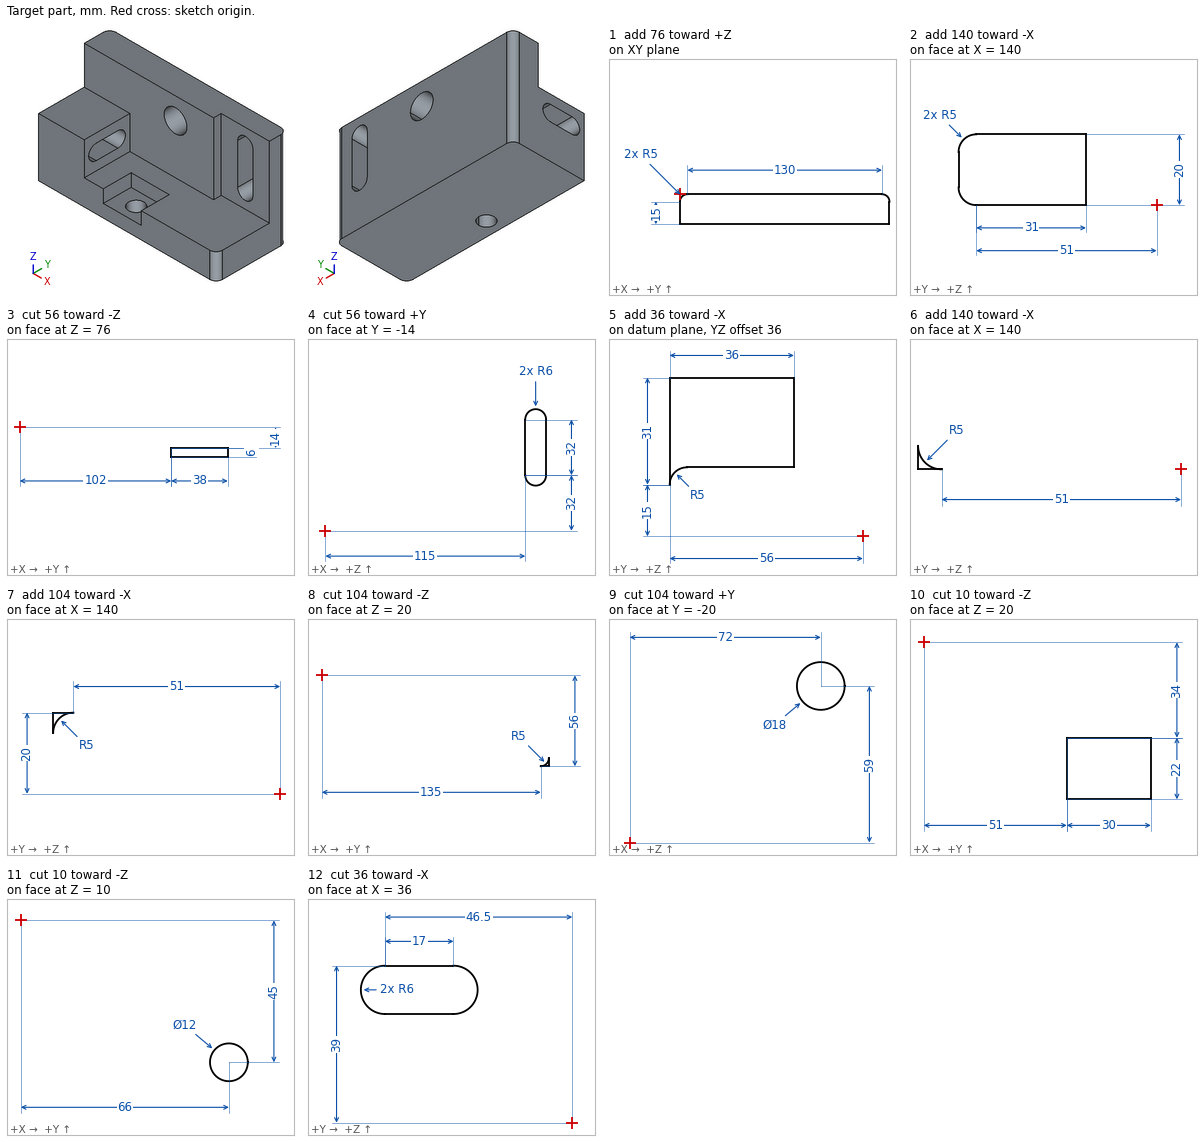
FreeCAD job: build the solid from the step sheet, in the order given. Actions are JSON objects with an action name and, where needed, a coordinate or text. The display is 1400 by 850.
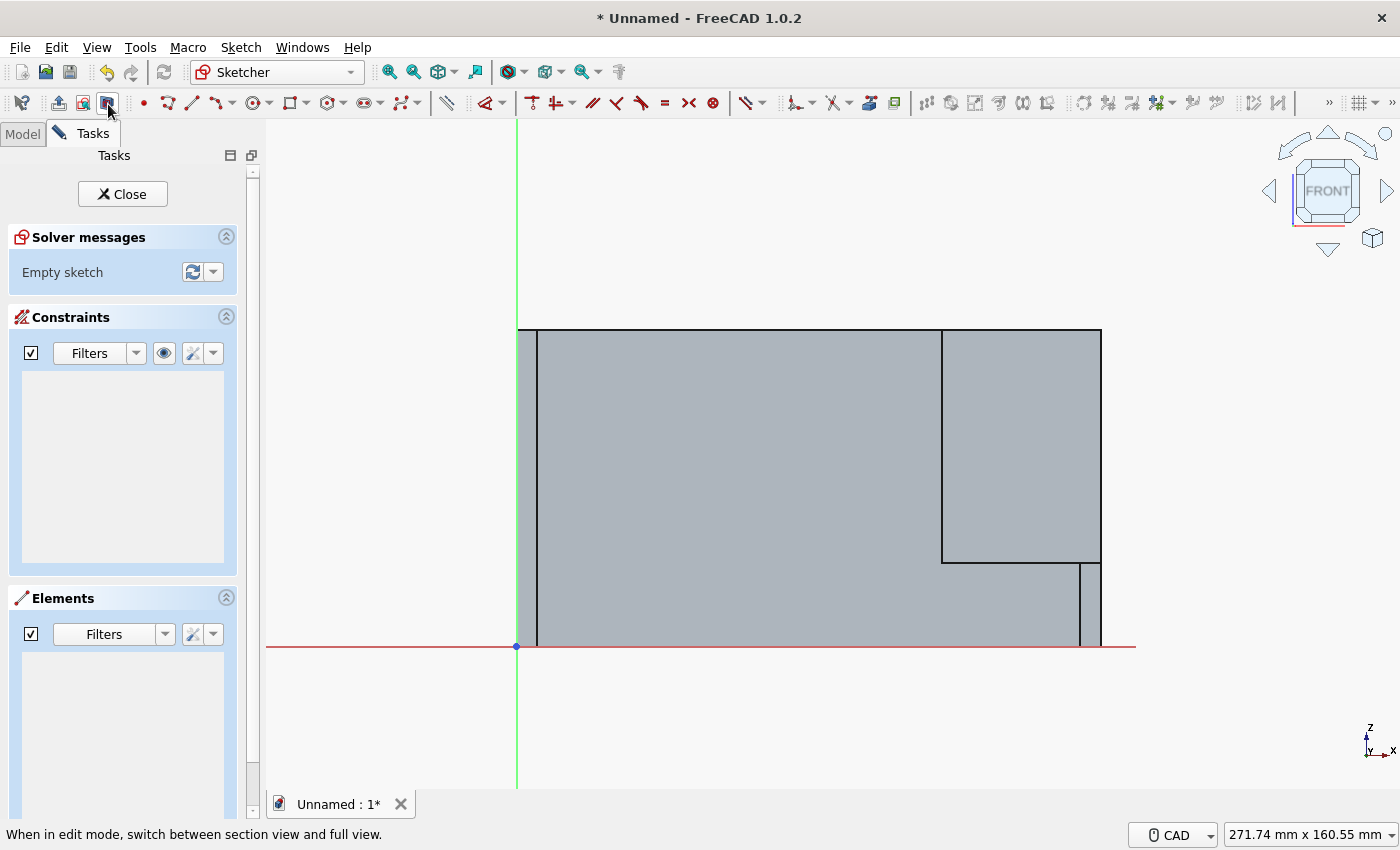
{"action": "scroll", "coordinate": [1231, 440], "scroll_direction": "up", "scroll_amount": 4}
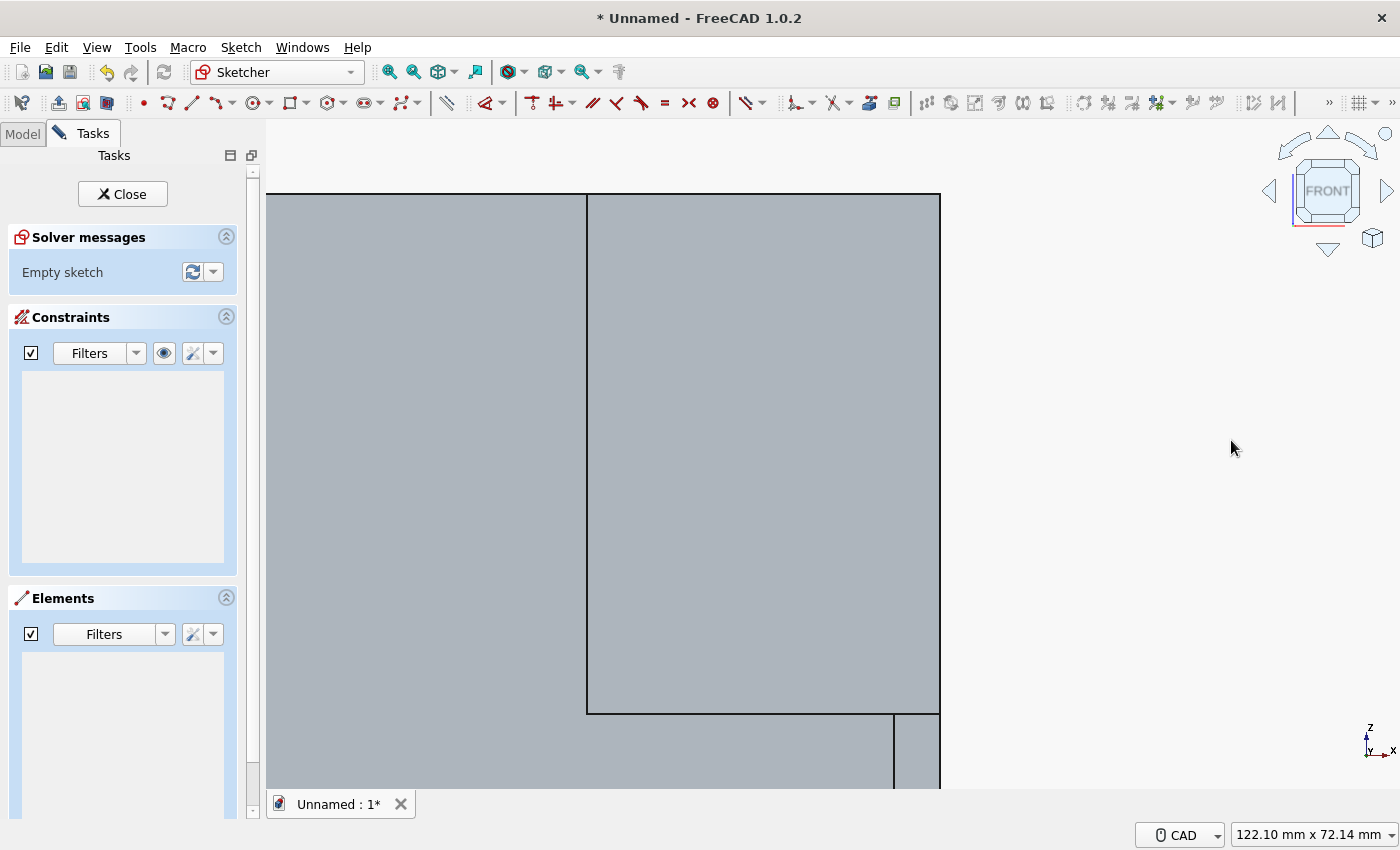
{"action": "left_click", "coordinate": [364, 104]}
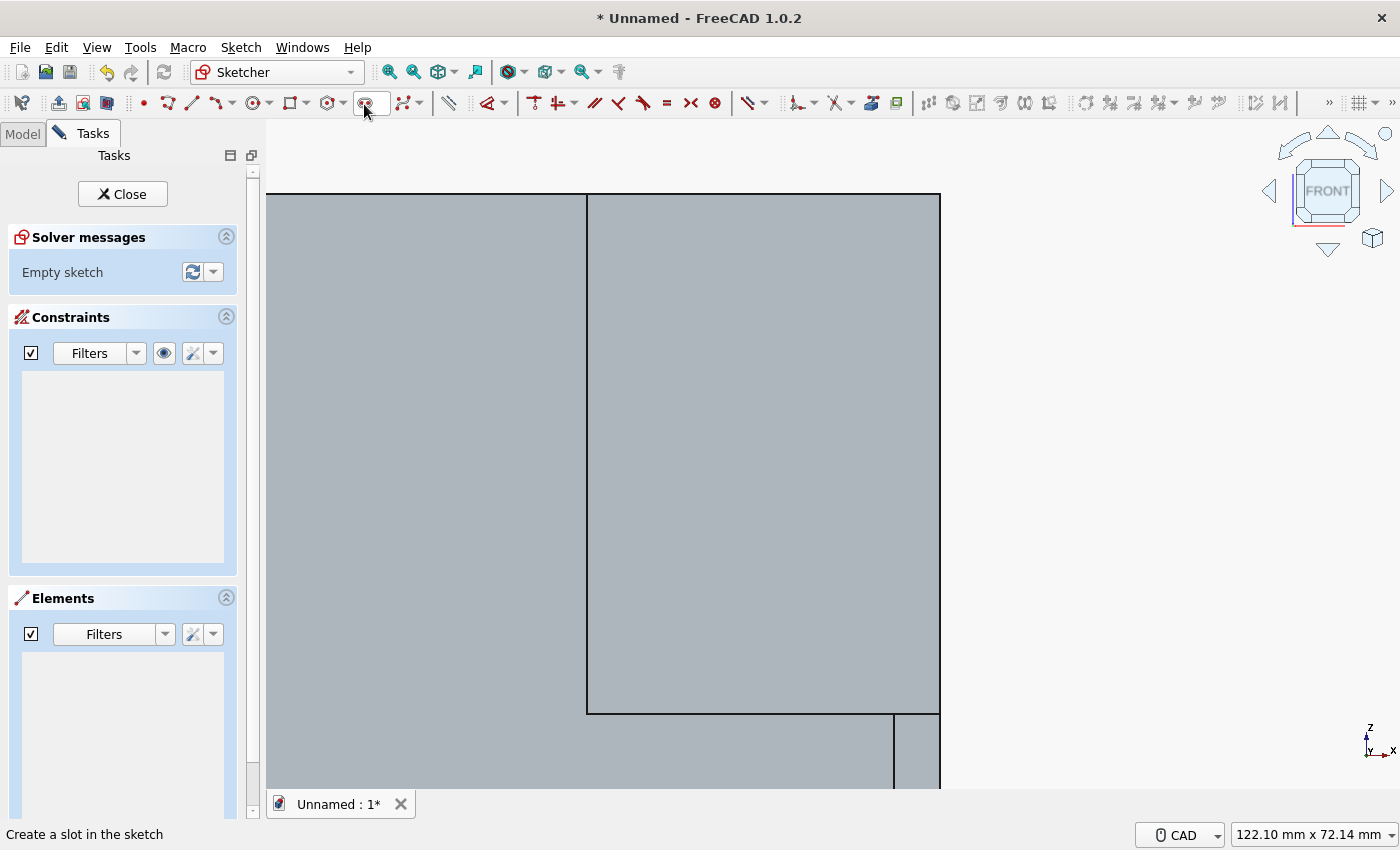
{"action": "left_click", "coordinate": [764, 602]}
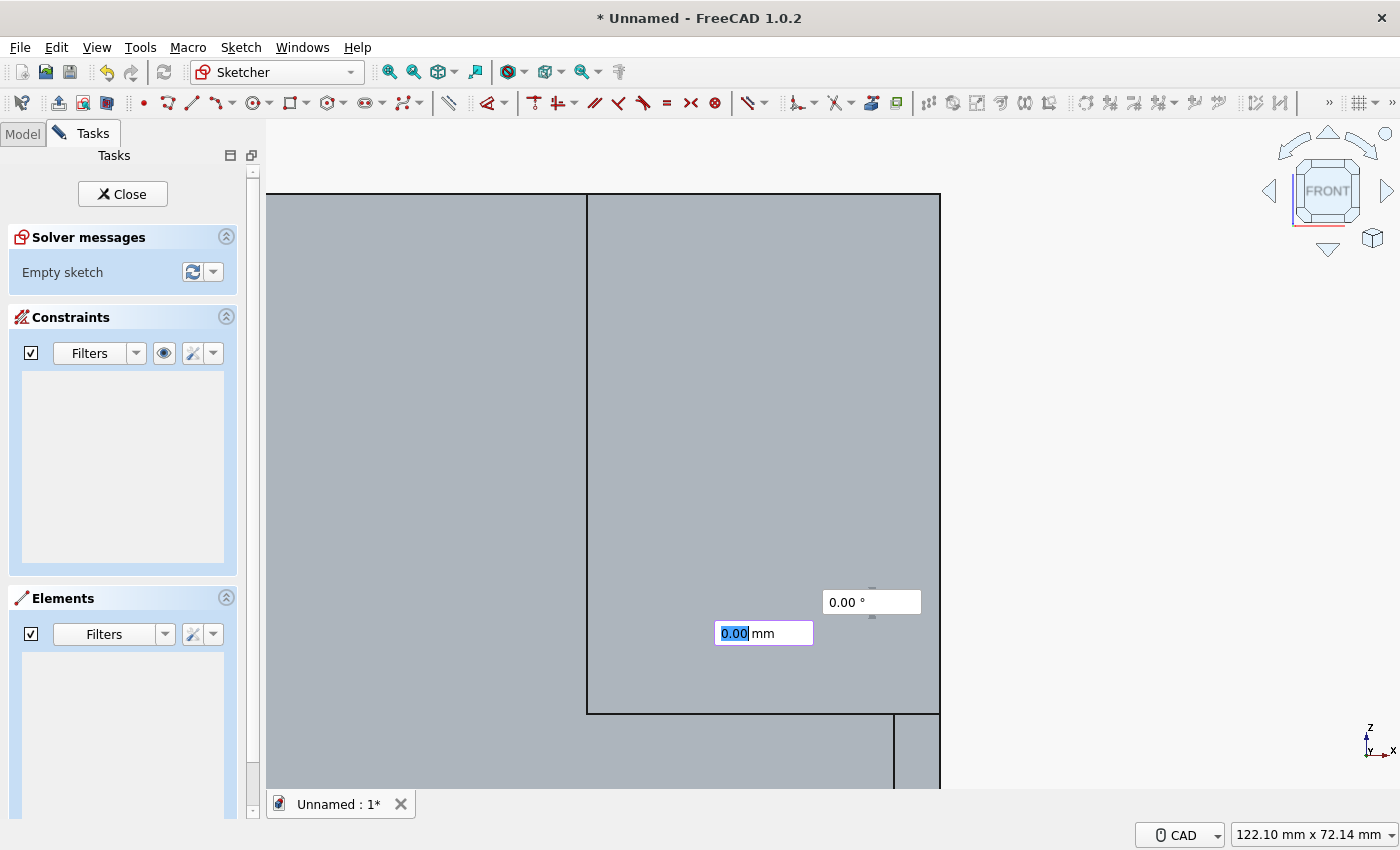
{"action": "left_click", "coordinate": [764, 305]}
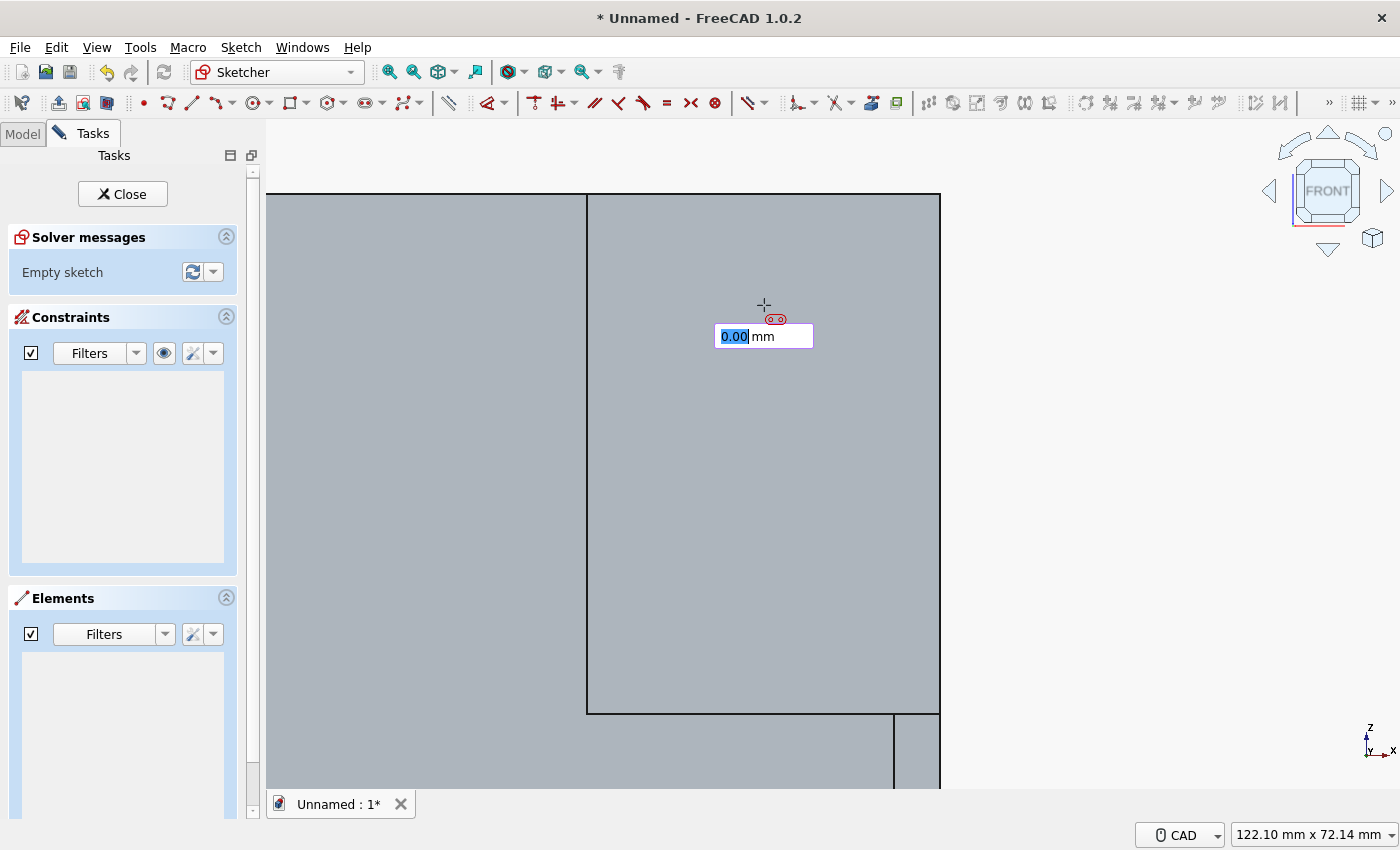
{"action": "left_click", "coordinate": [708, 454]}
{"action": "key", "text": "Escape"}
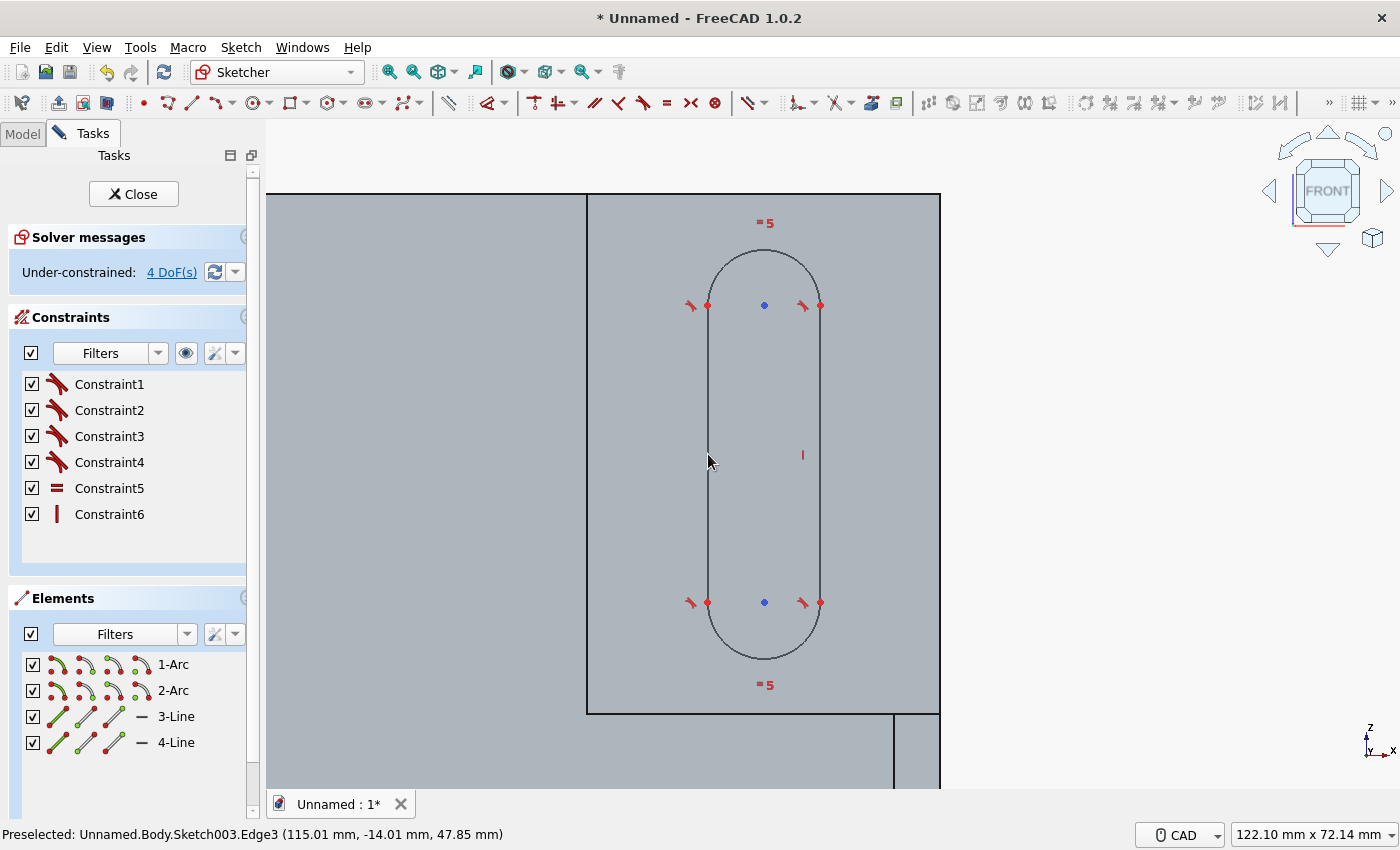
{"action": "left_click", "coordinate": [488, 104]}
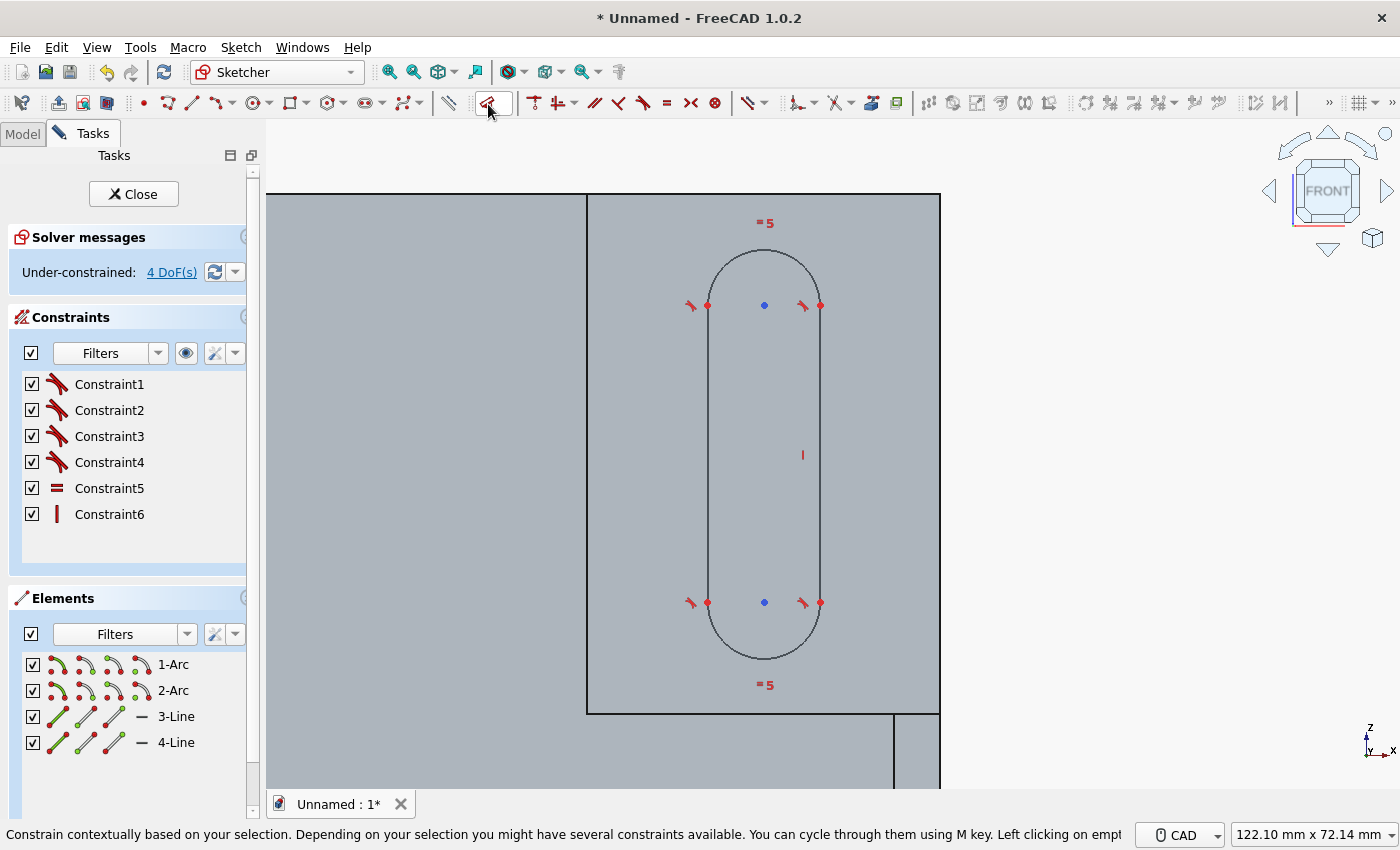
{"action": "left_click", "coordinate": [731, 648]}
{"action": "left_click", "coordinate": [712, 674]}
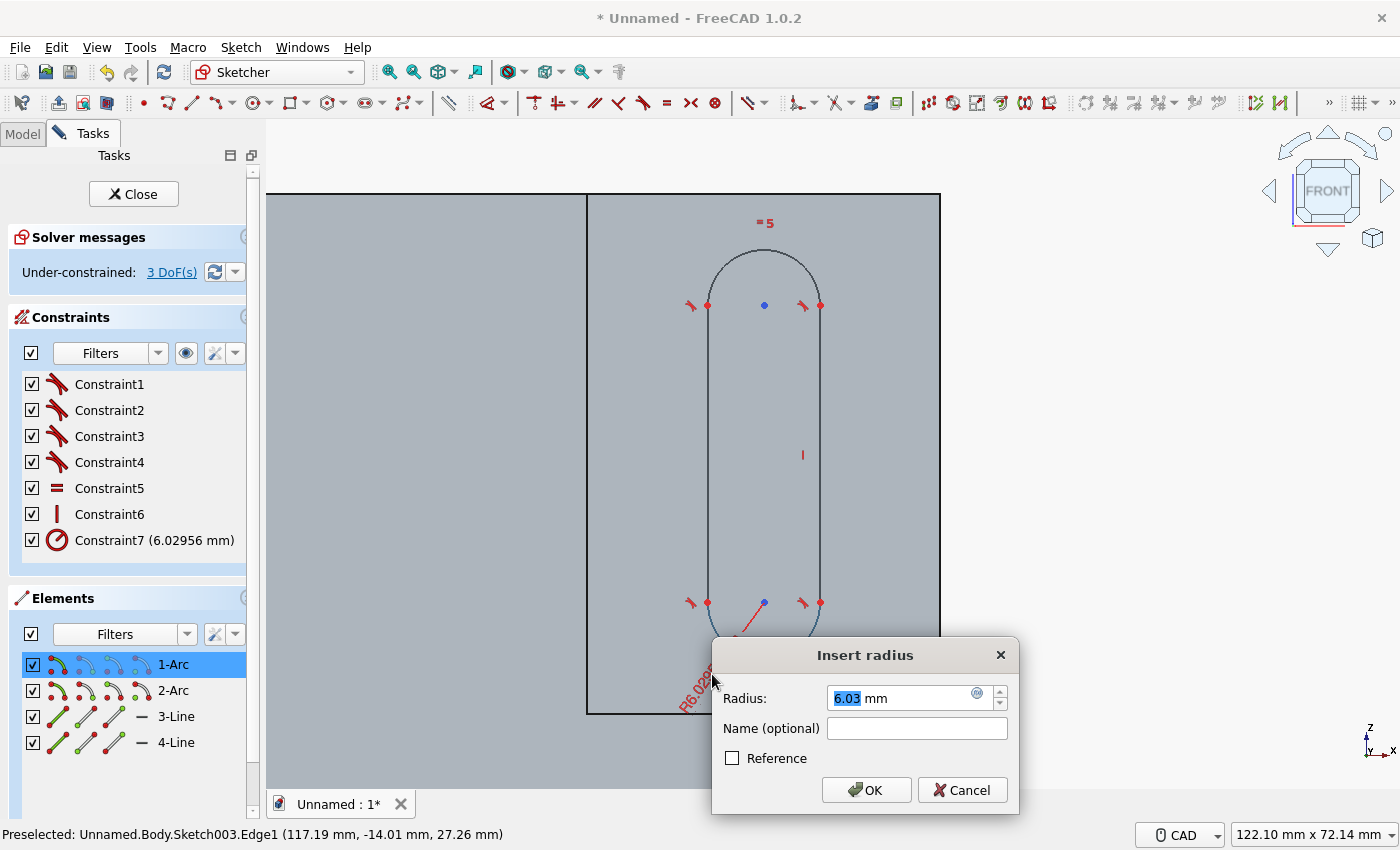
{"action": "type", "text": "6"}
{"action": "key", "text": "Return"}